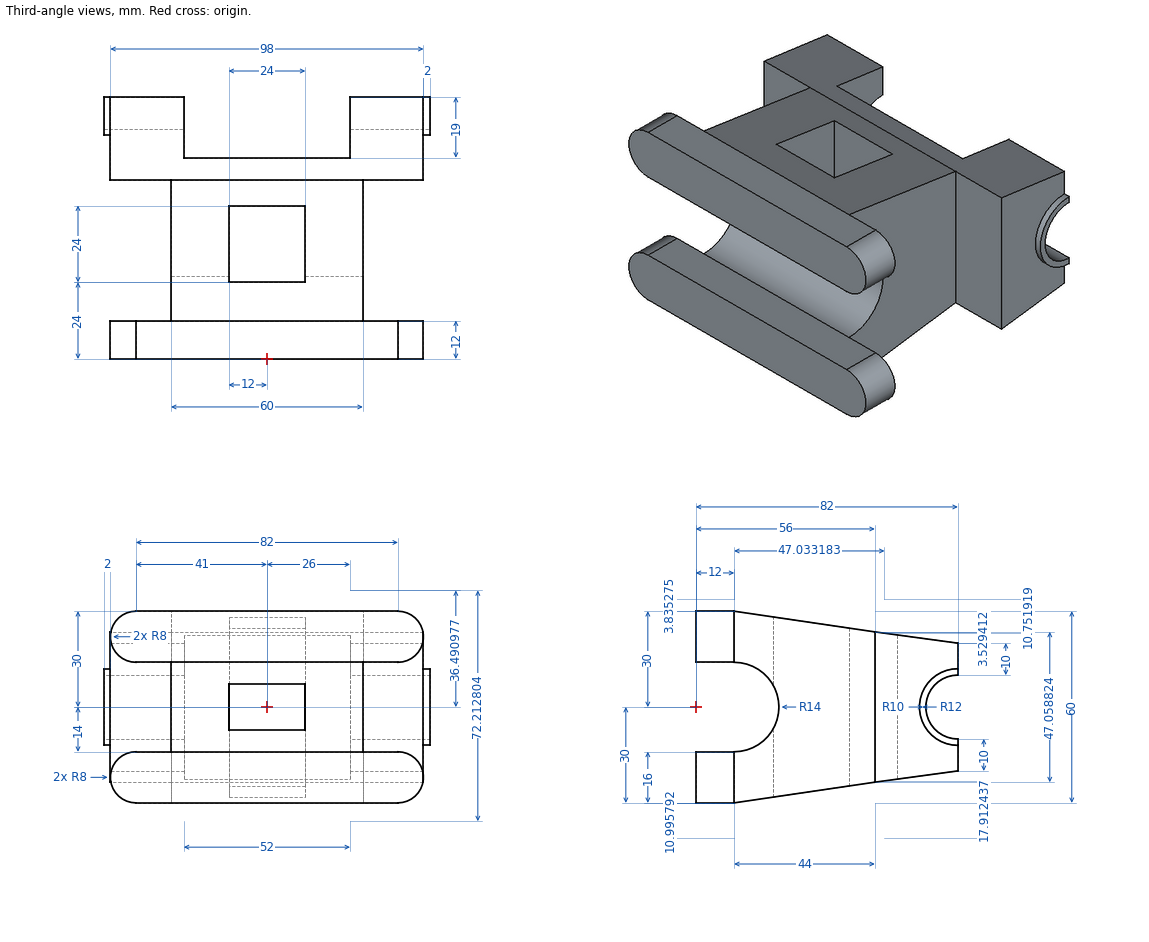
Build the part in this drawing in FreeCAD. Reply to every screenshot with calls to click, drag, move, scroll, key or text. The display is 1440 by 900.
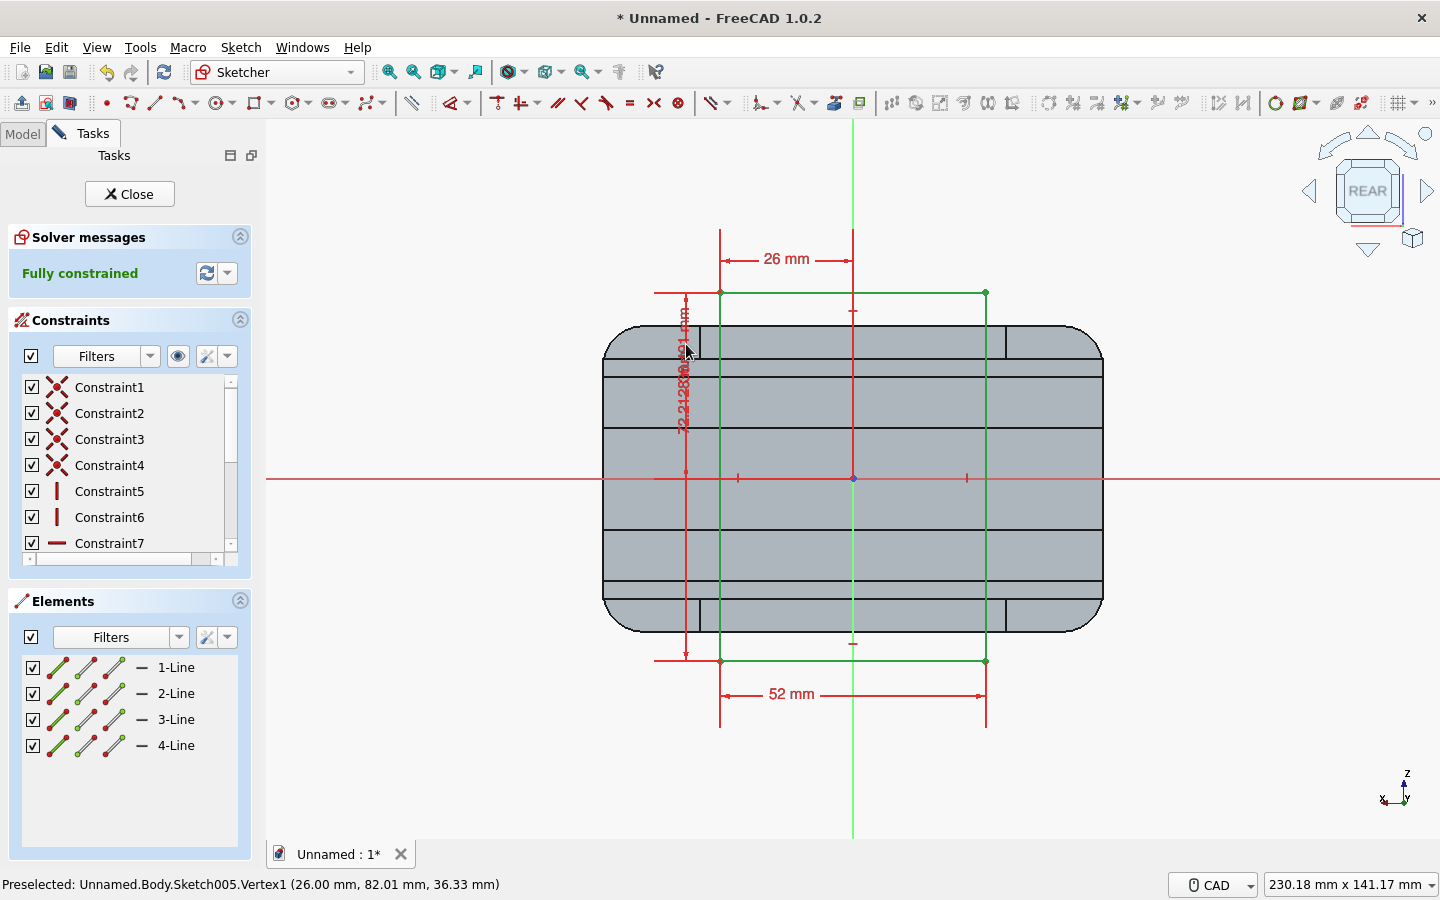
click(130, 194)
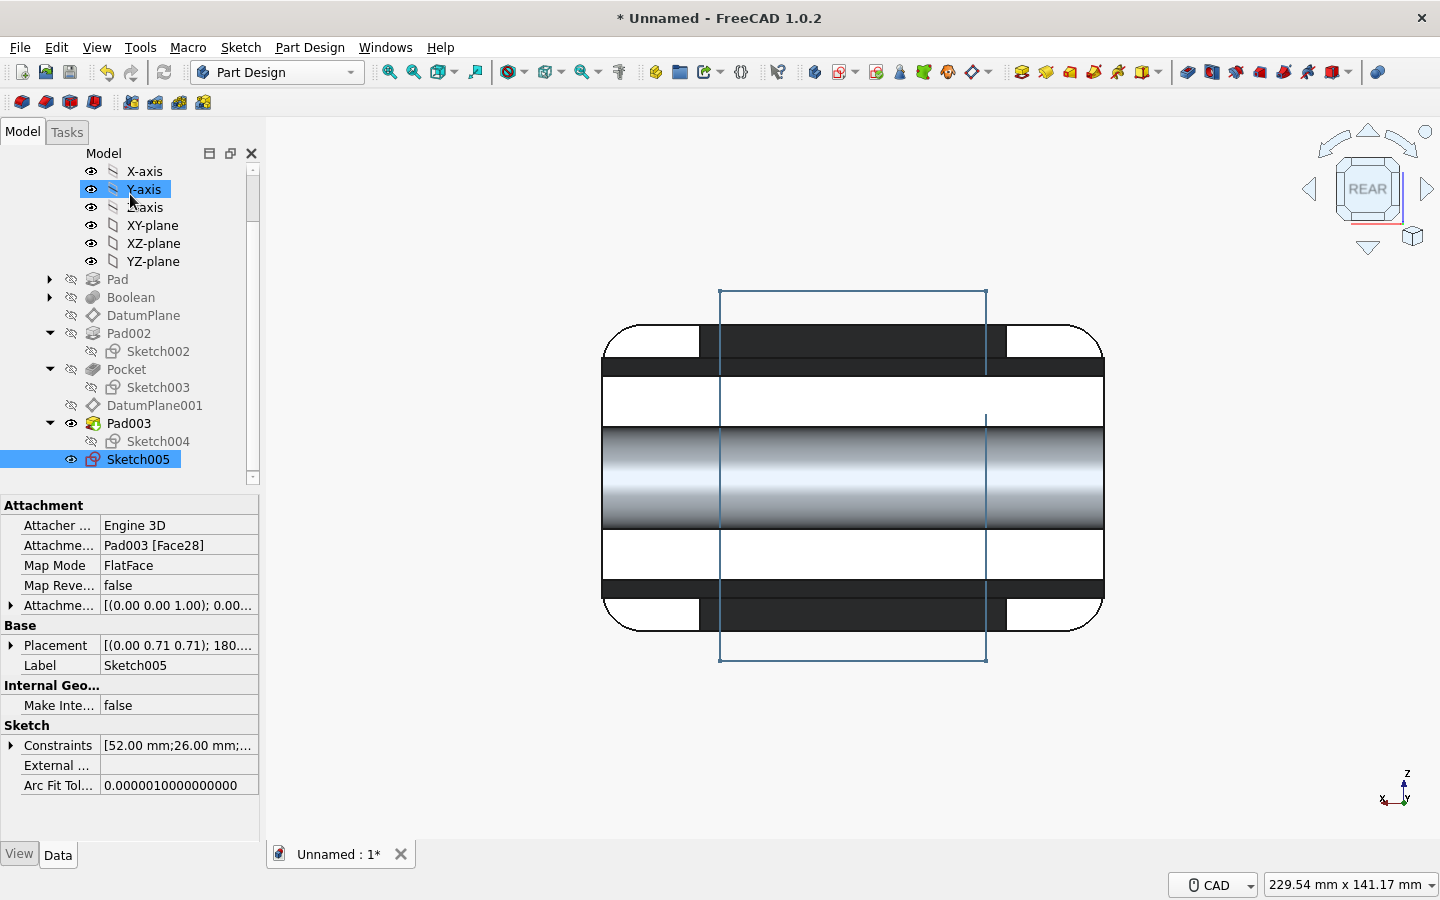
click(1188, 72)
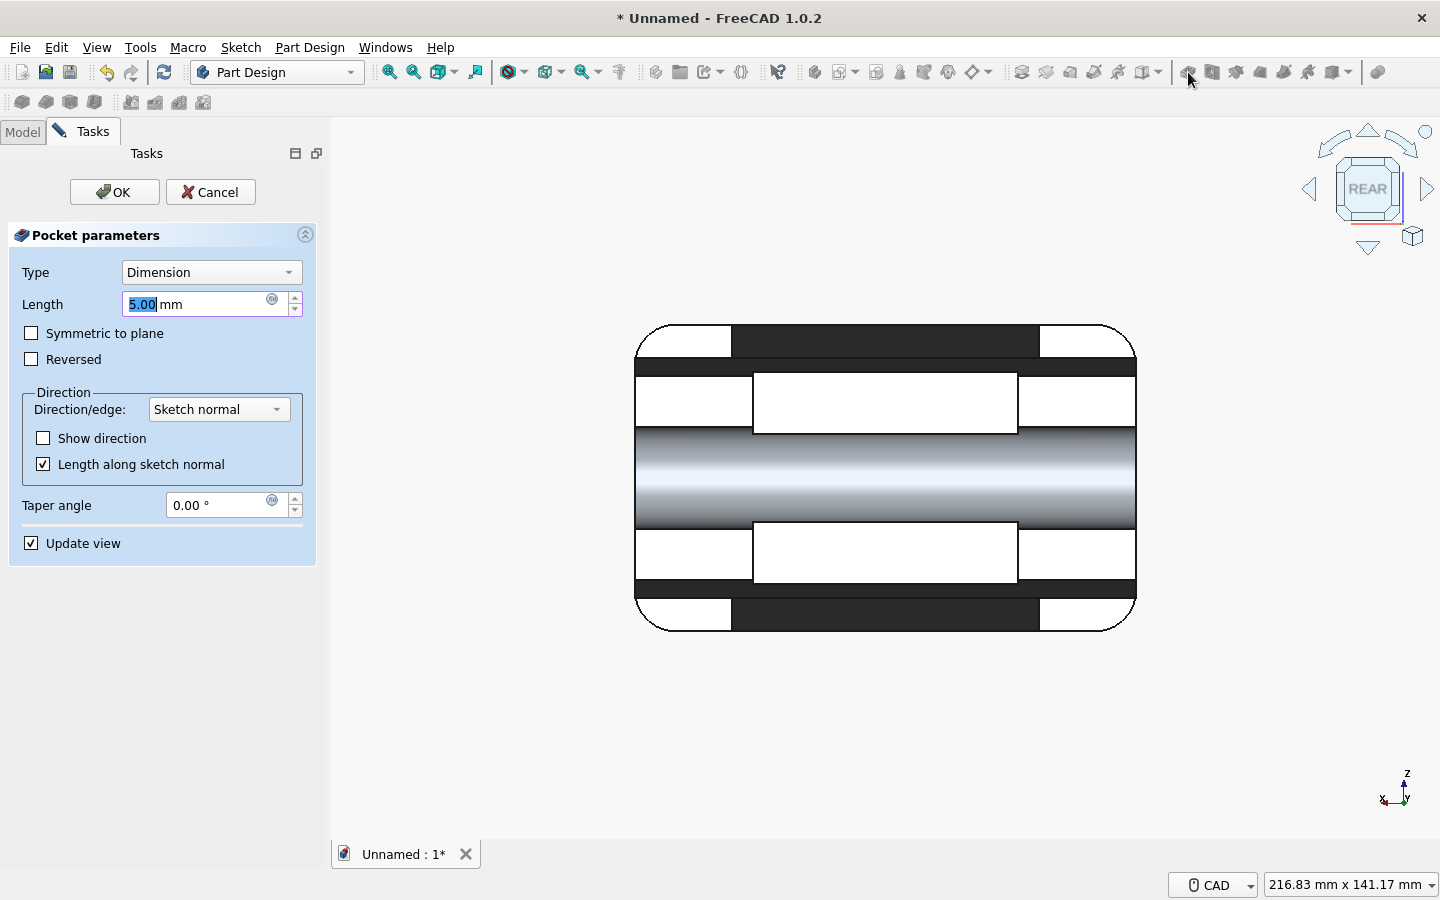
text(19)
key(Tab)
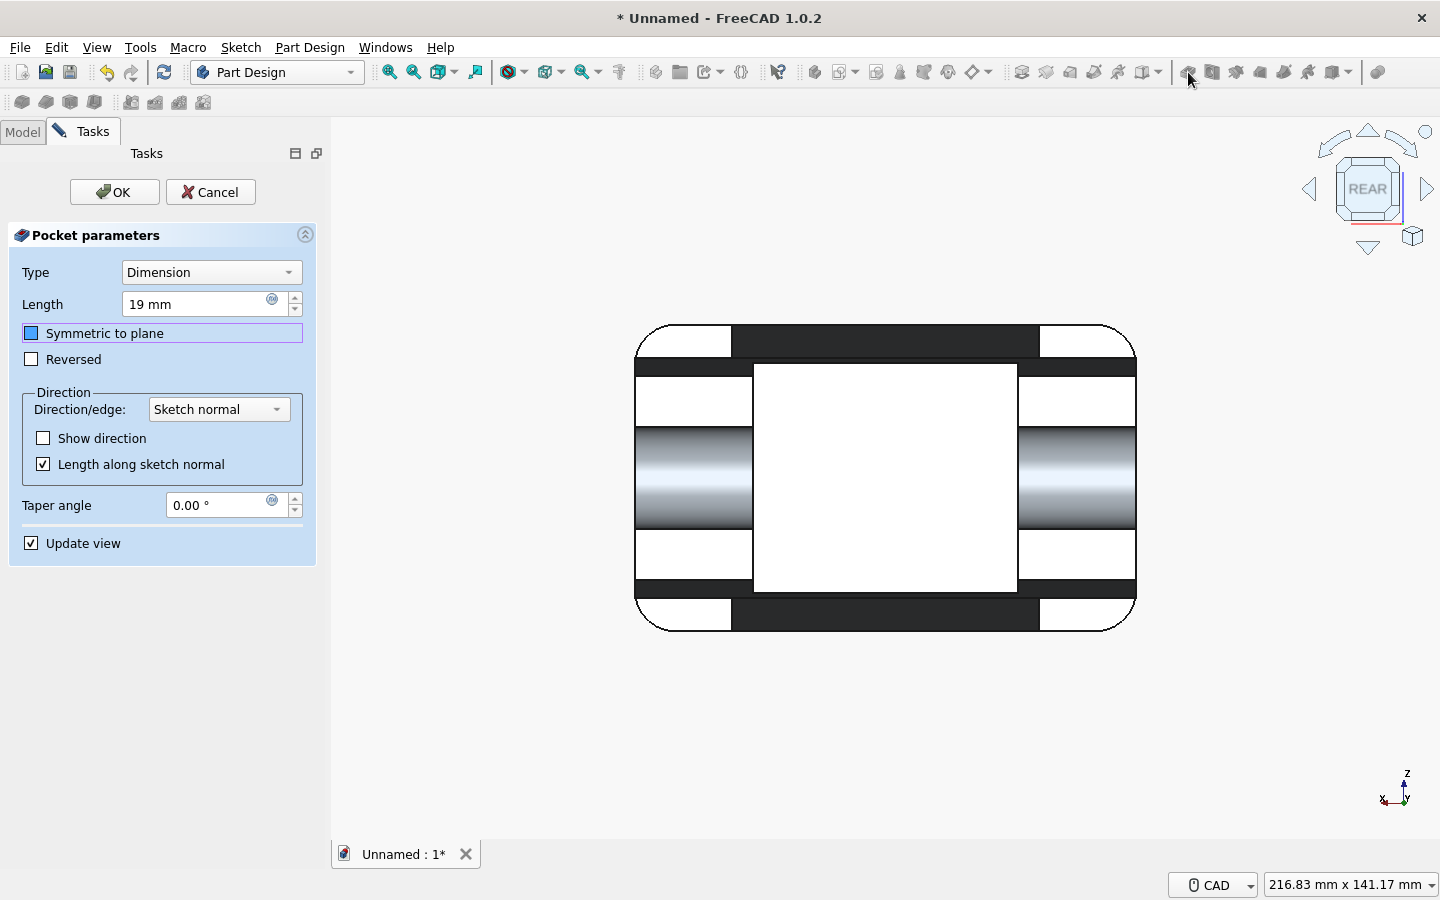
click(115, 192)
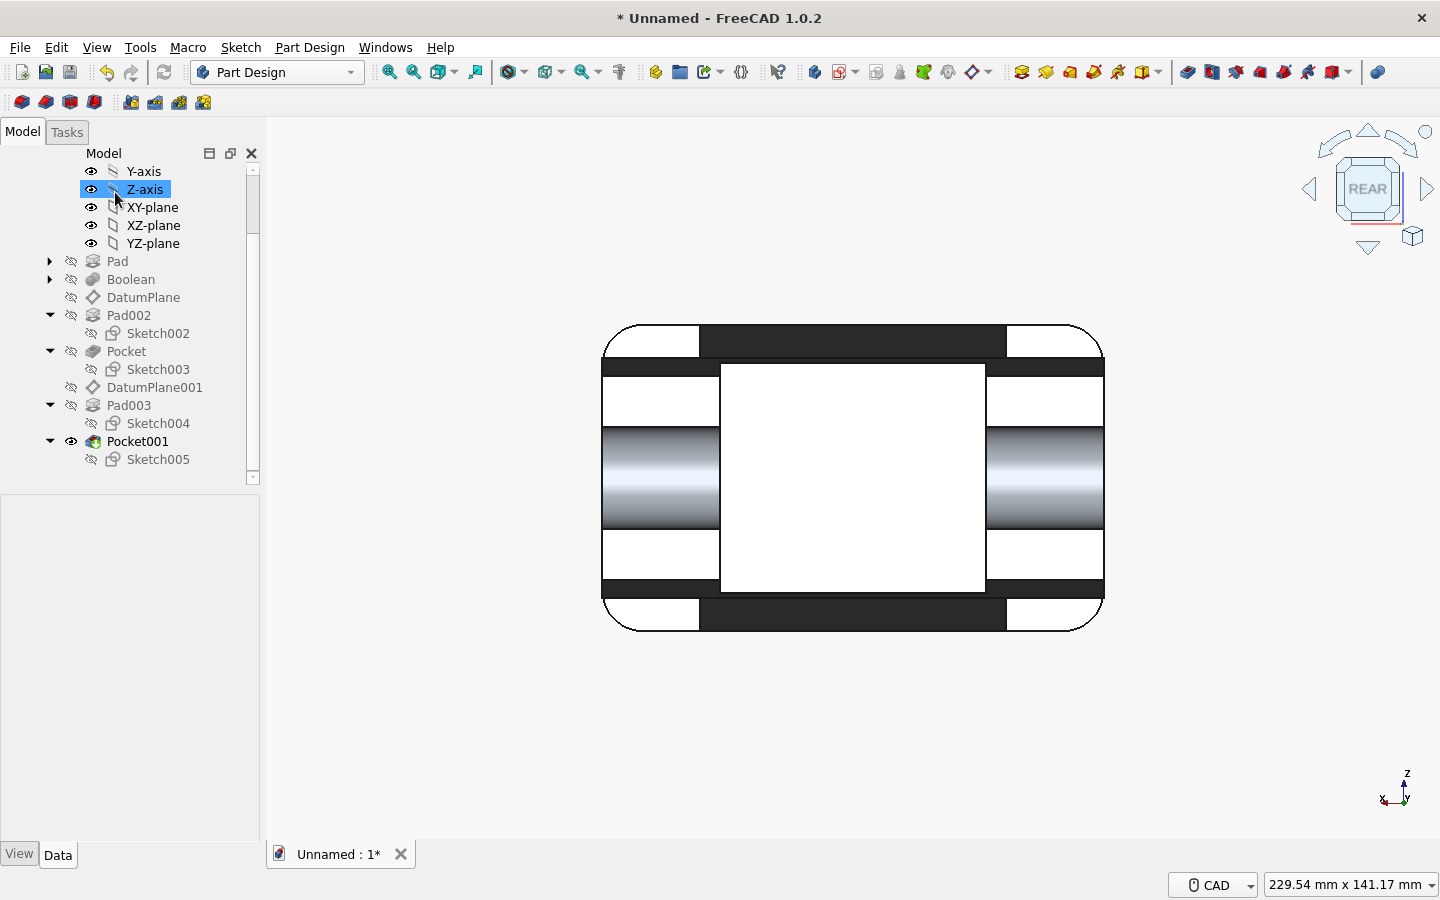
click(390, 72)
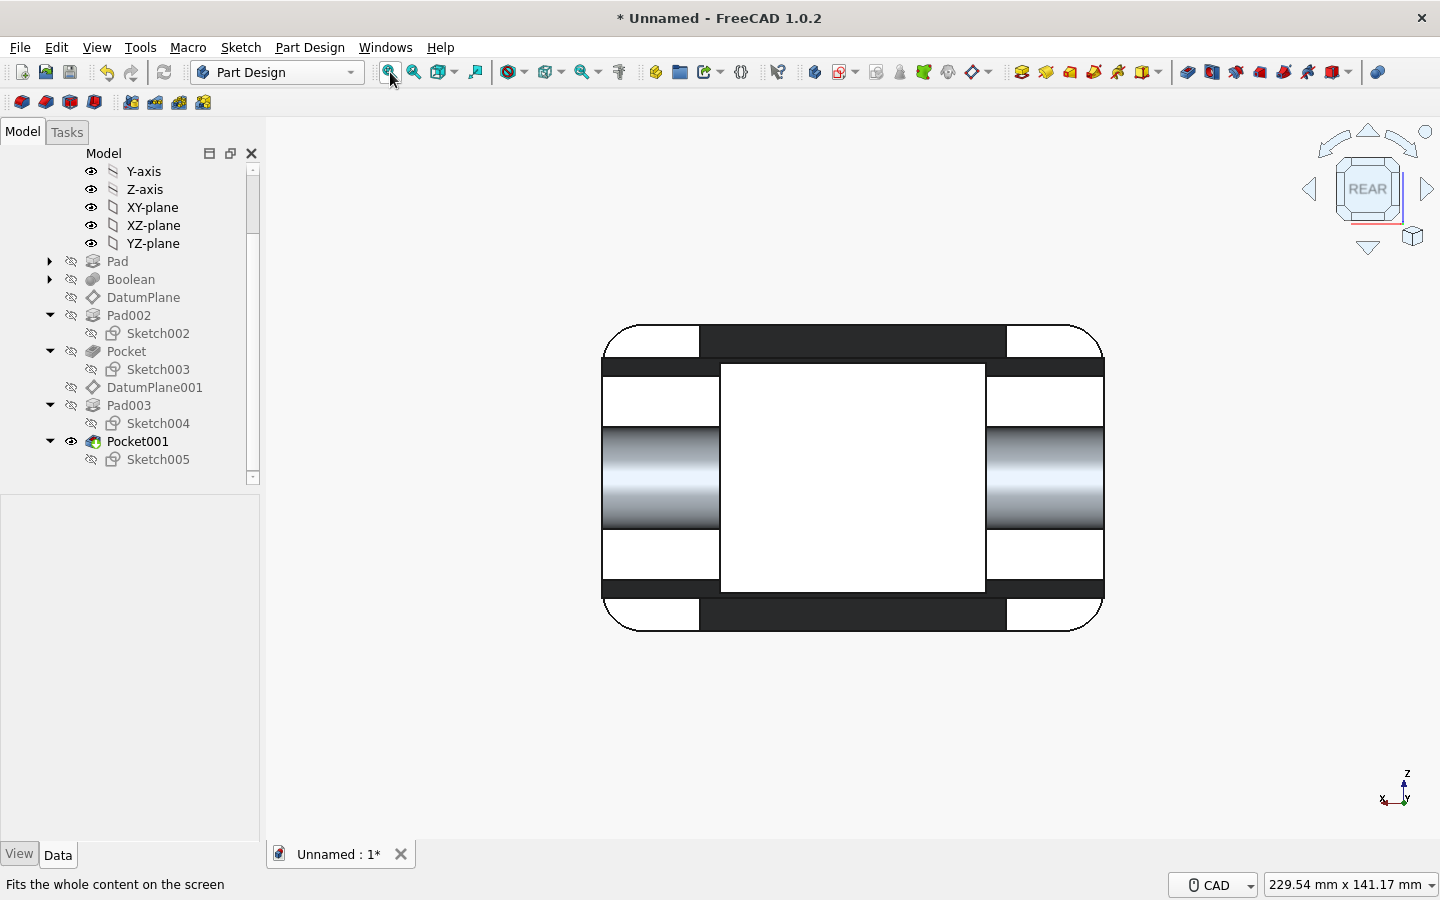
key(5)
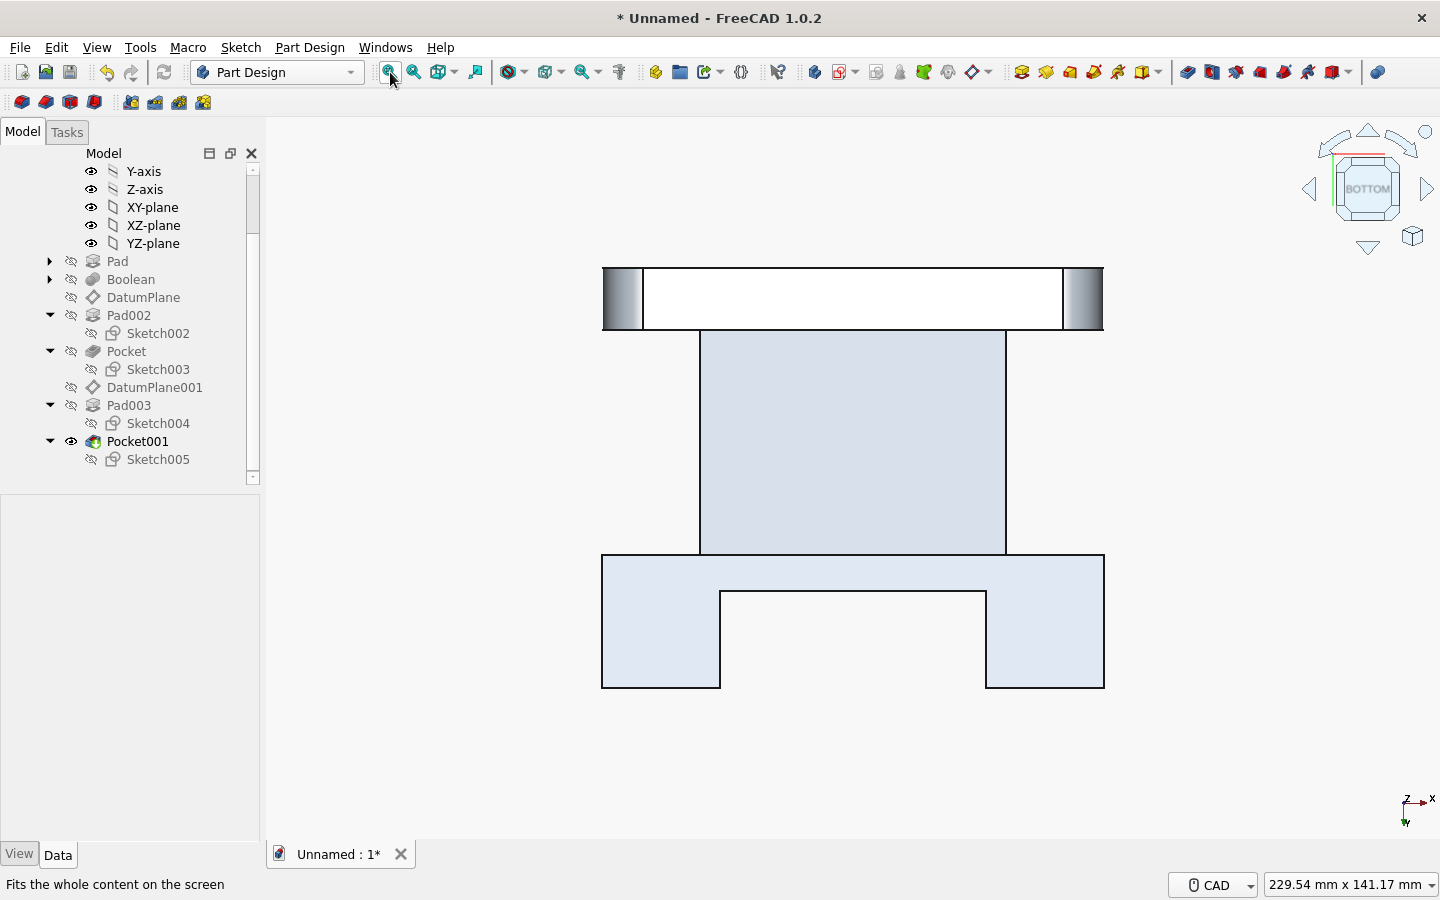
click(973, 298)